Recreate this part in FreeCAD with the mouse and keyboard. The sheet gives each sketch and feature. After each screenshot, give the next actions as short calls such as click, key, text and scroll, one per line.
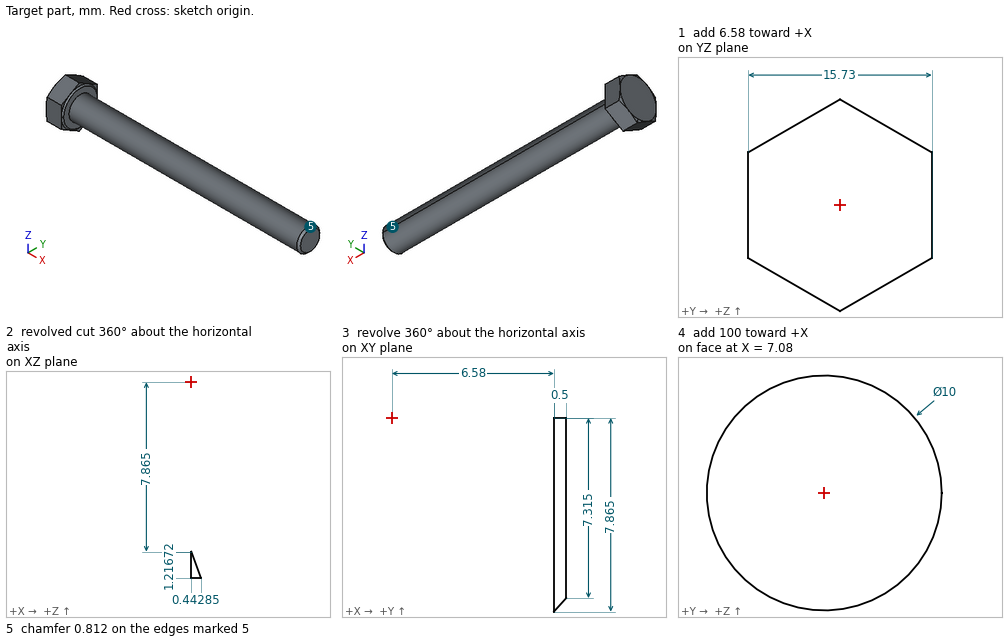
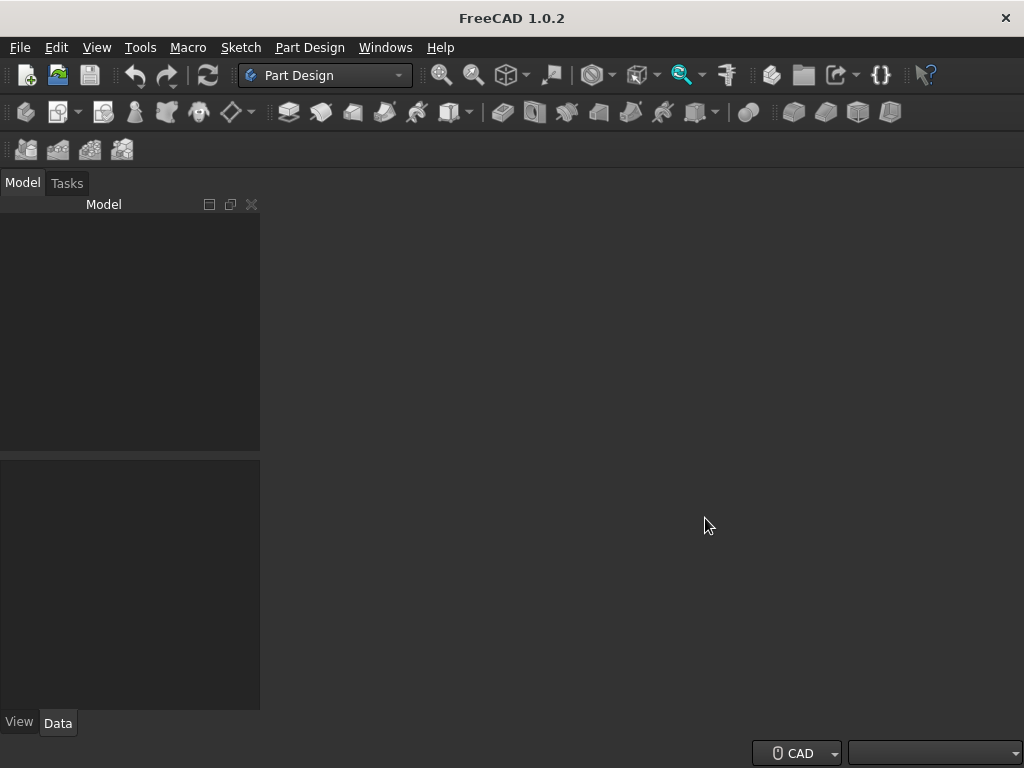
click(26, 76)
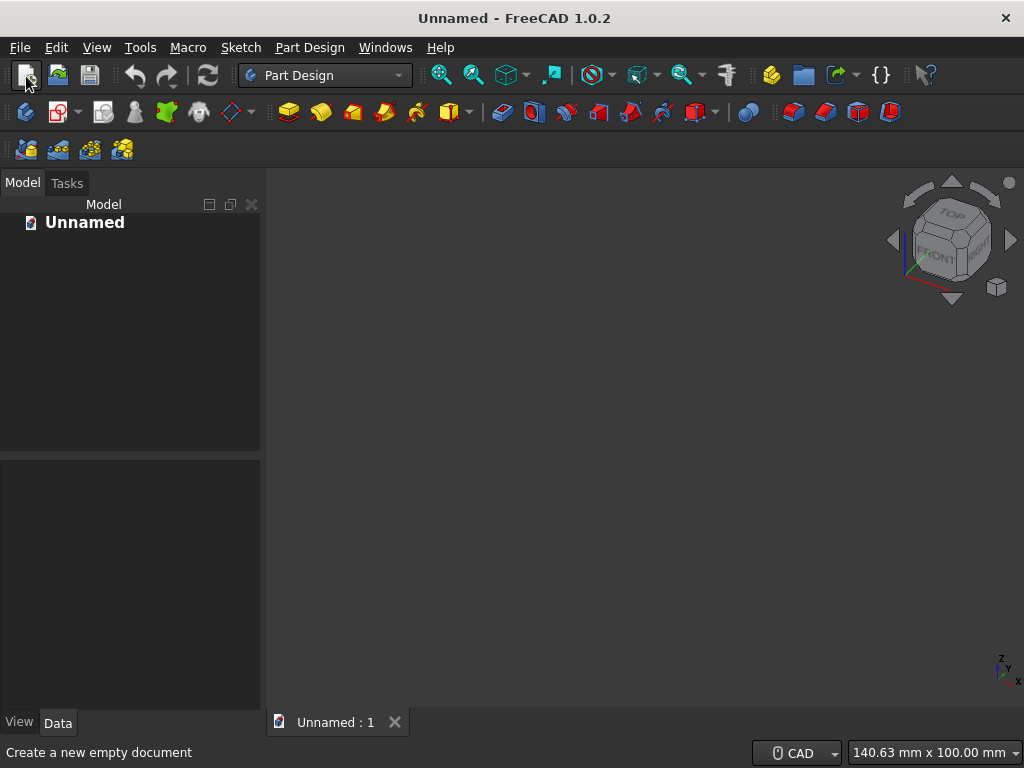
click(58, 112)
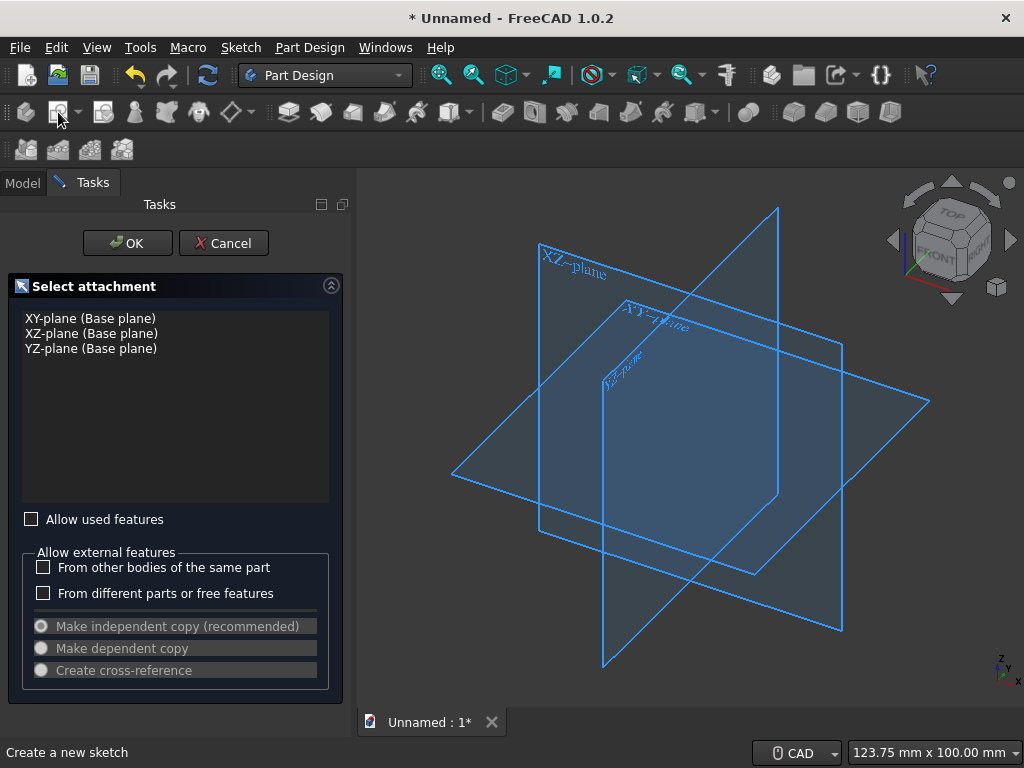
click(82, 348)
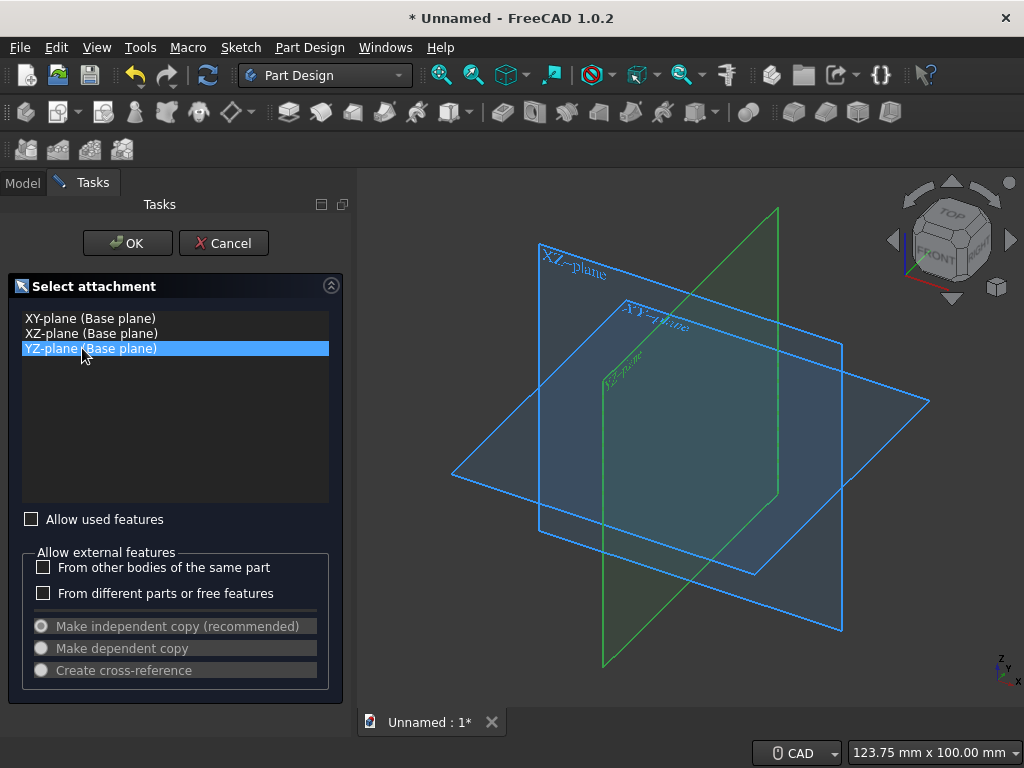
click(128, 243)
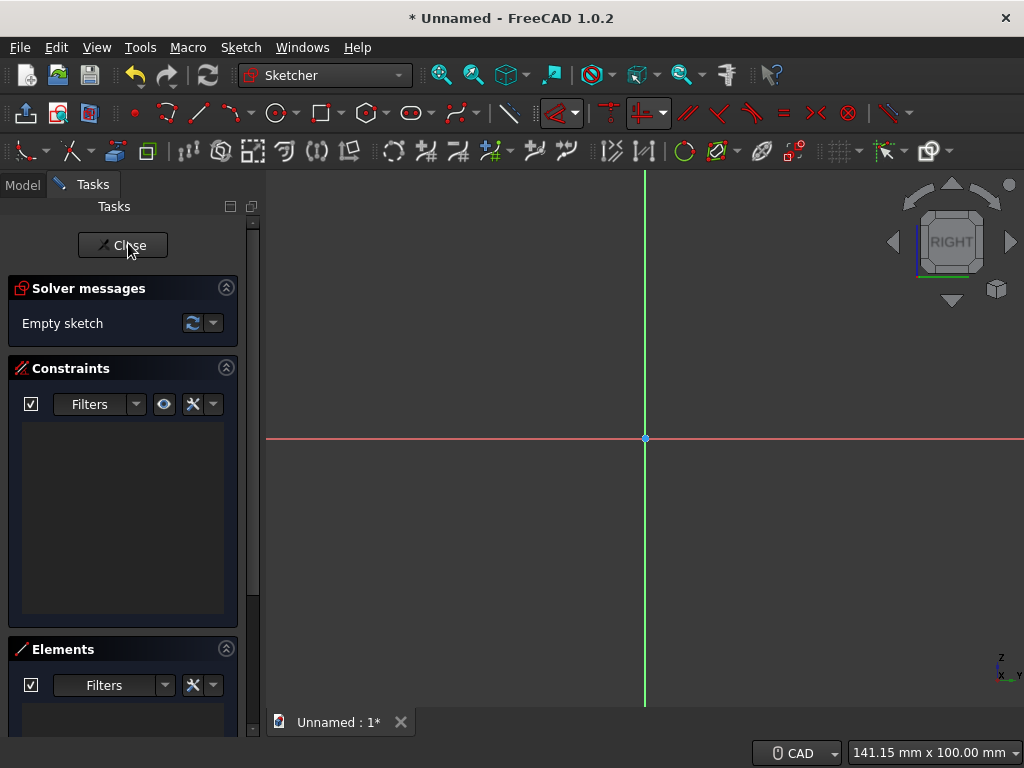
scroll(675, 438, up, 6)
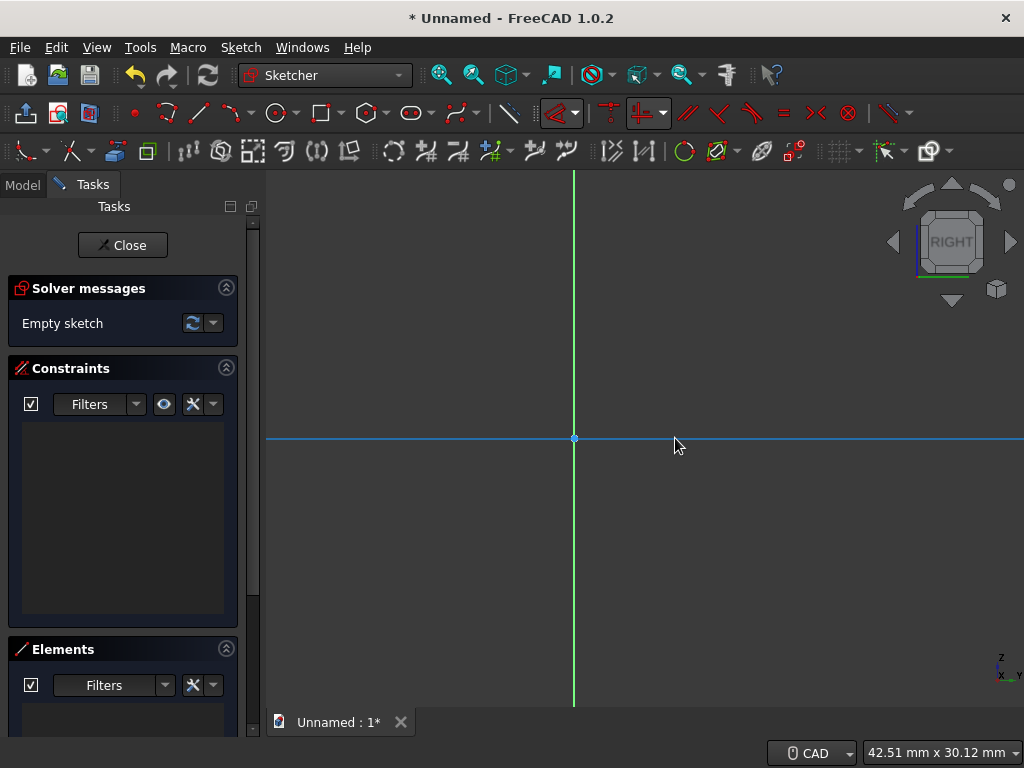
click(366, 114)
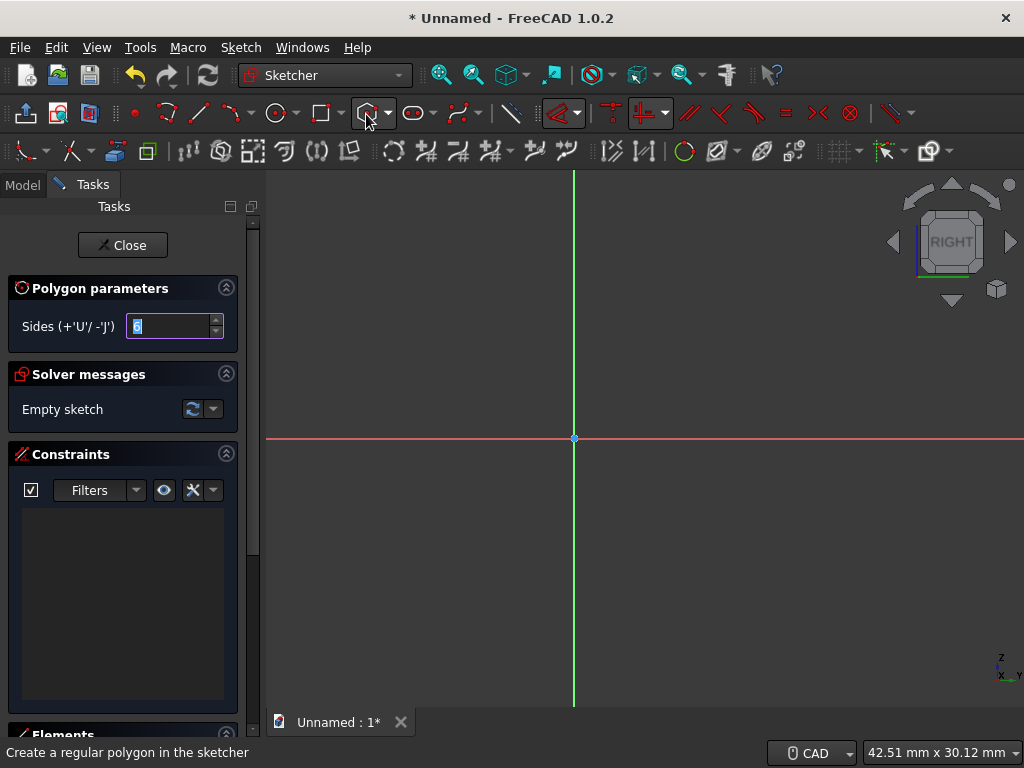
click(574, 438)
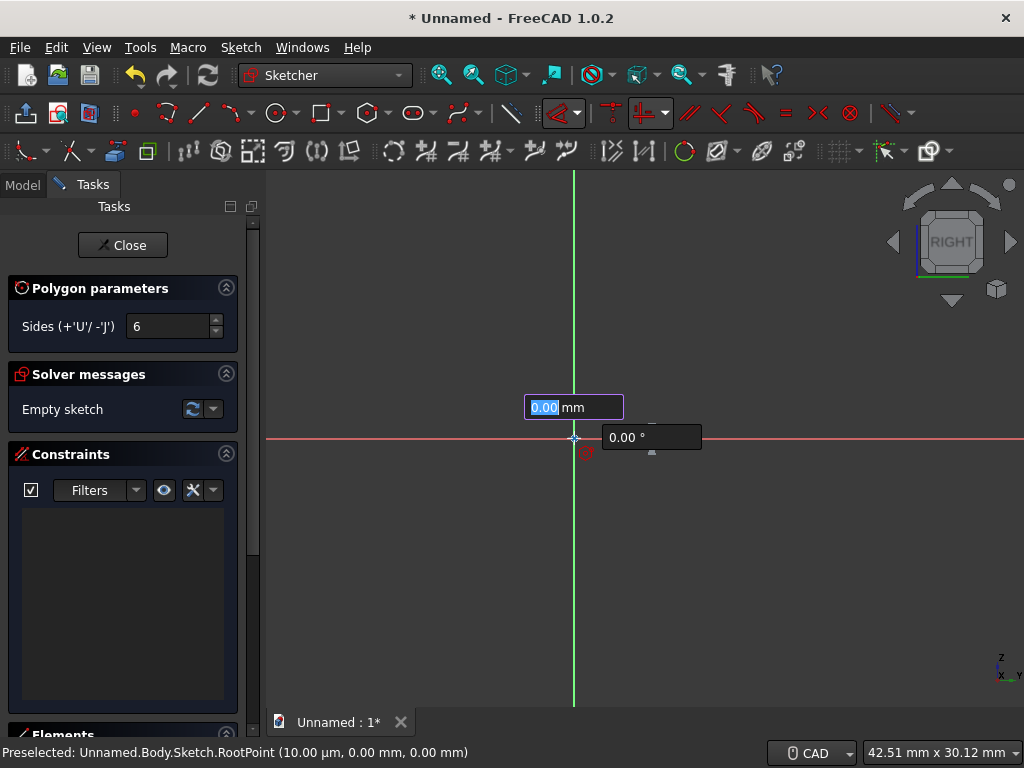
click(574, 600)
key(Escape)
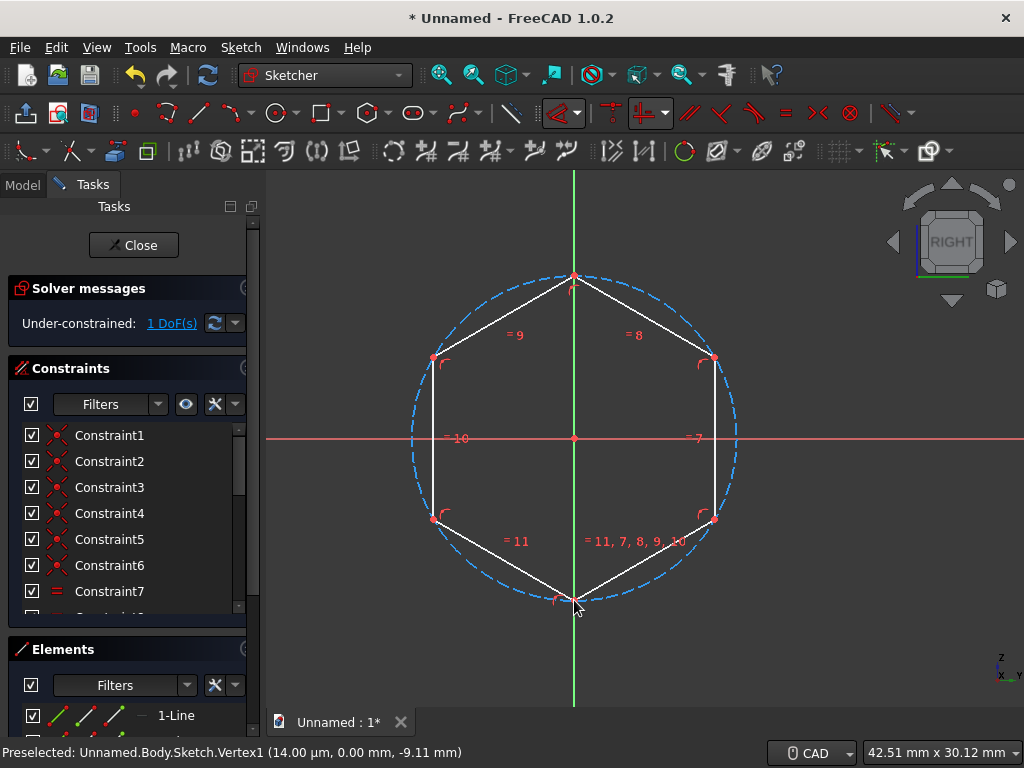
key(d)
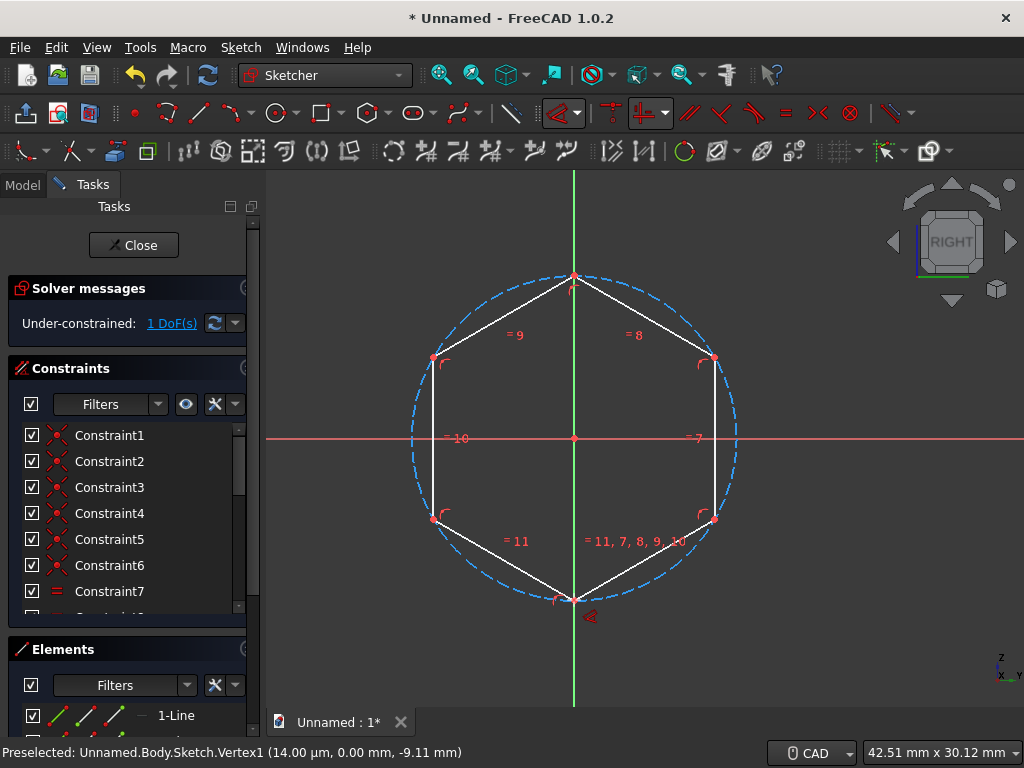
click(433, 357)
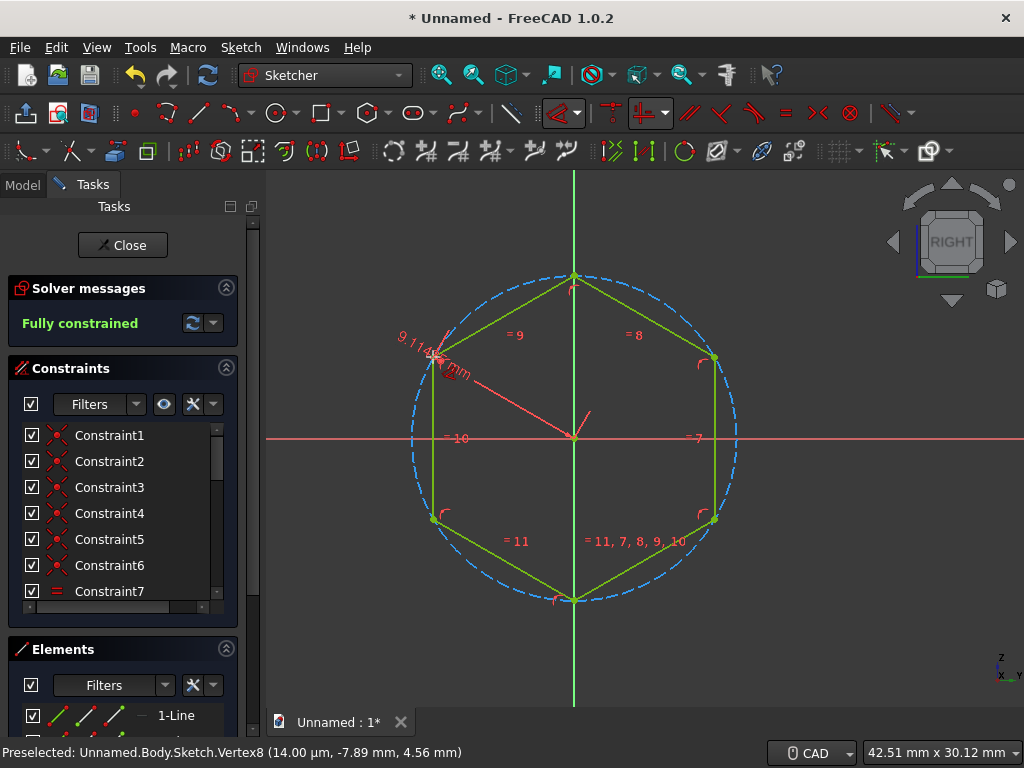
click(715, 520)
click(509, 275)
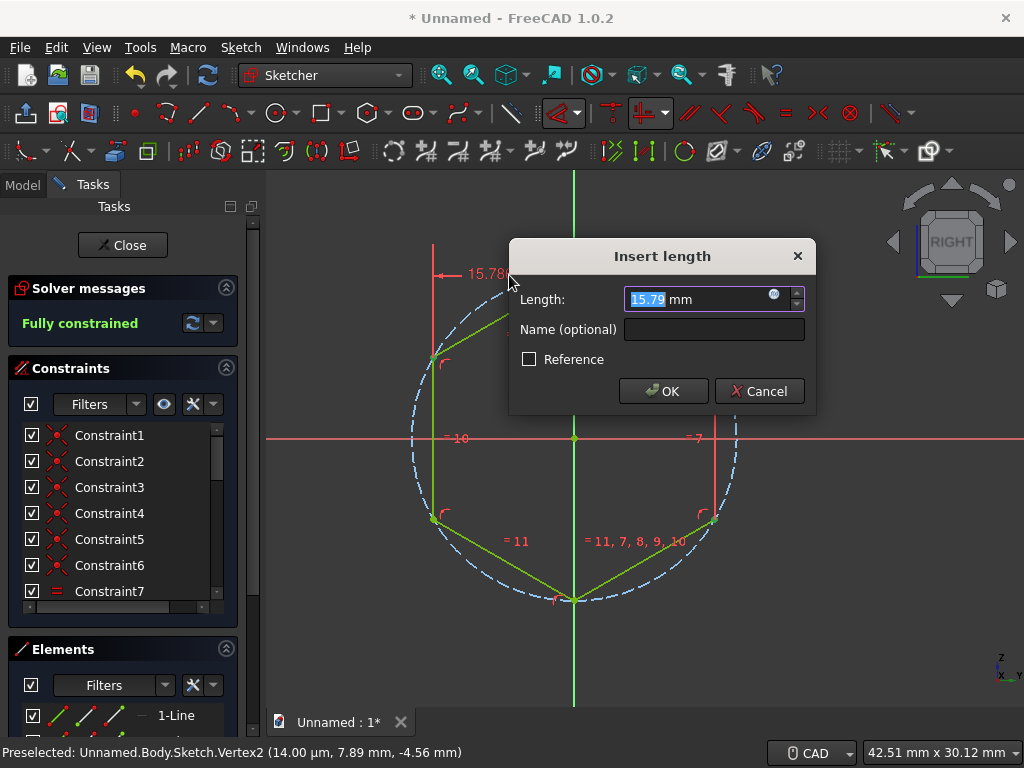
text(15.73)
key(Return)
key(Escape)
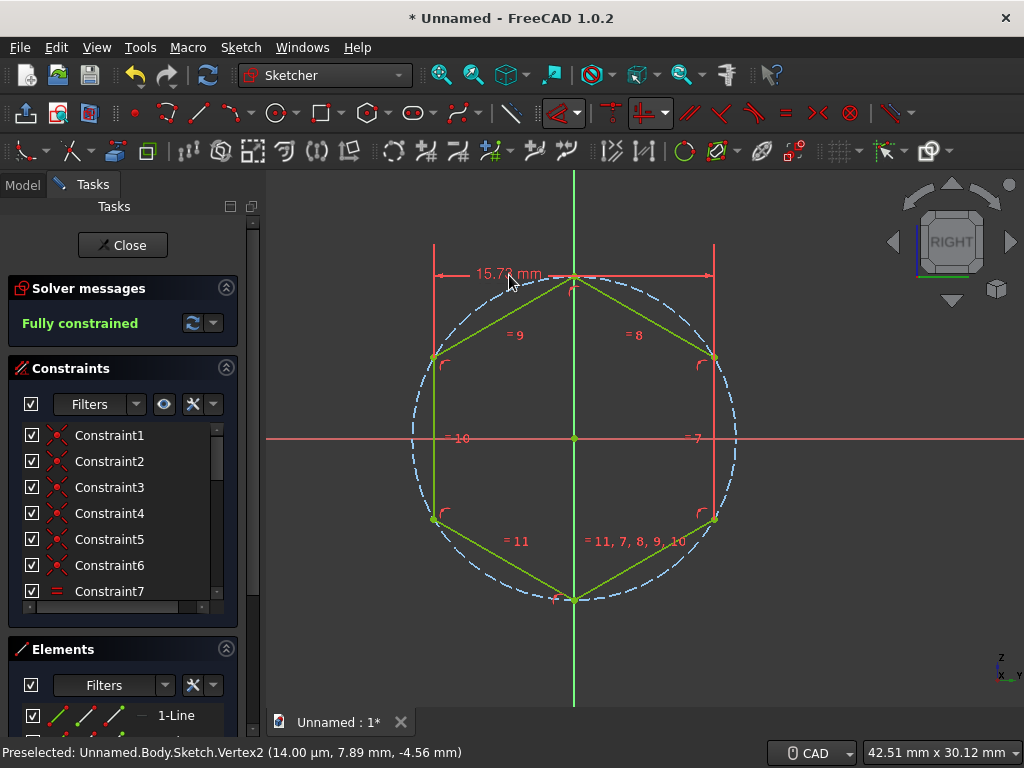
click(123, 245)